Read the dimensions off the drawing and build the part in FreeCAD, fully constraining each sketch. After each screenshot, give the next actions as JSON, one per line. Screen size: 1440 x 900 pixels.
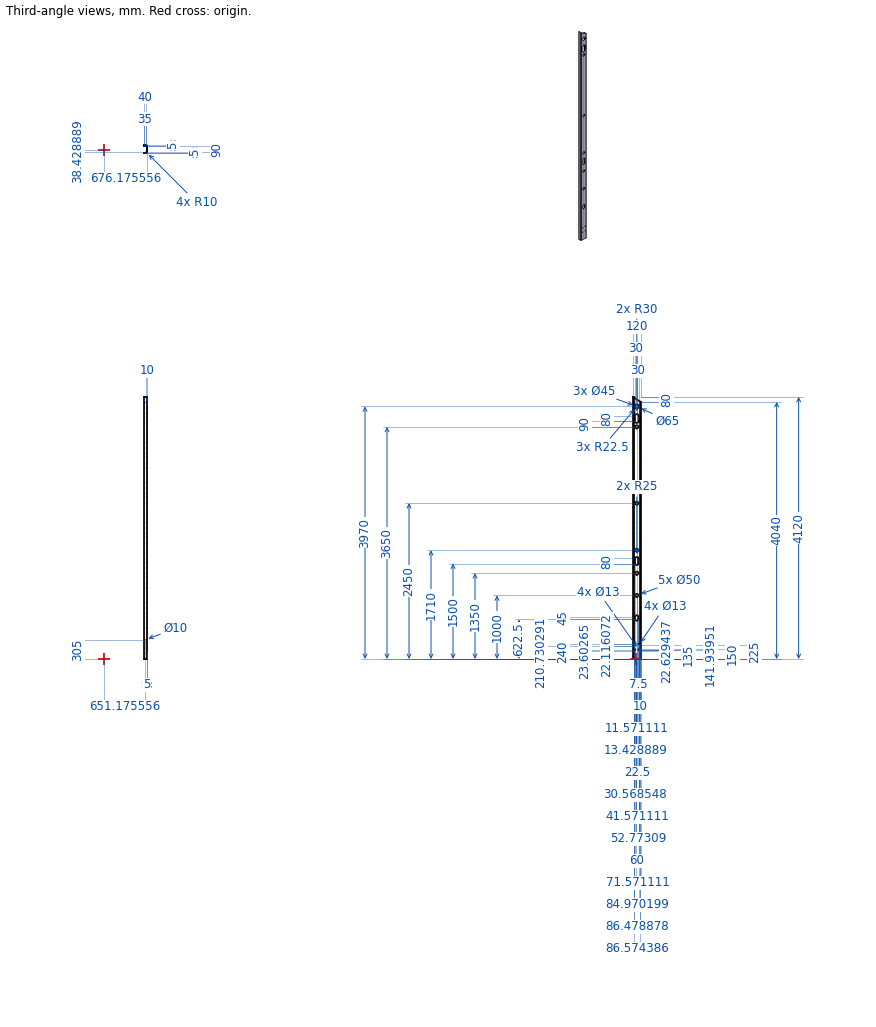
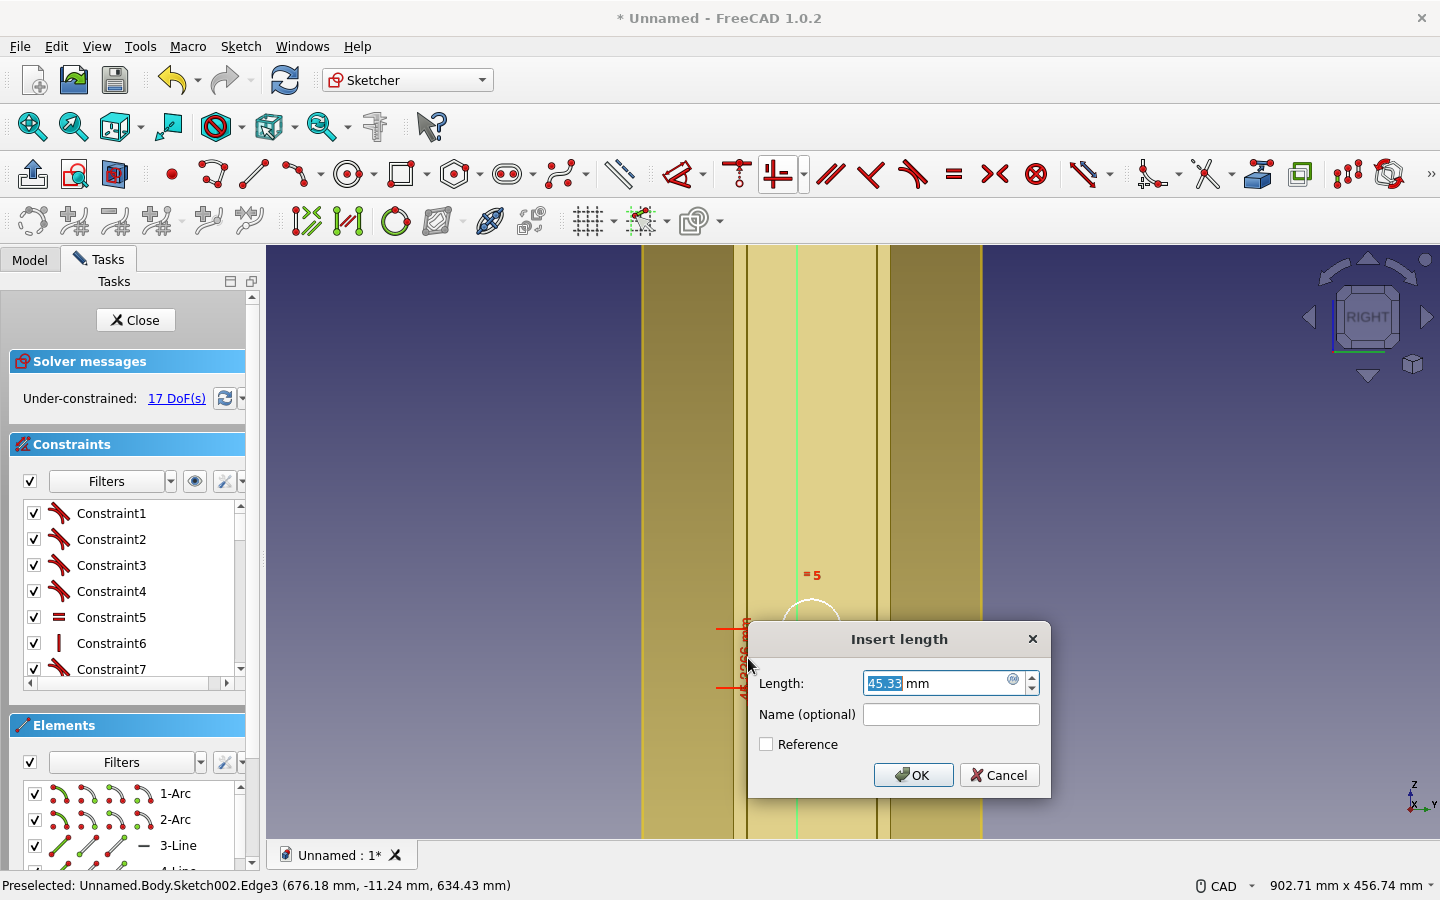
{"action": "type", "text": "45"}
{"action": "key", "text": "Return"}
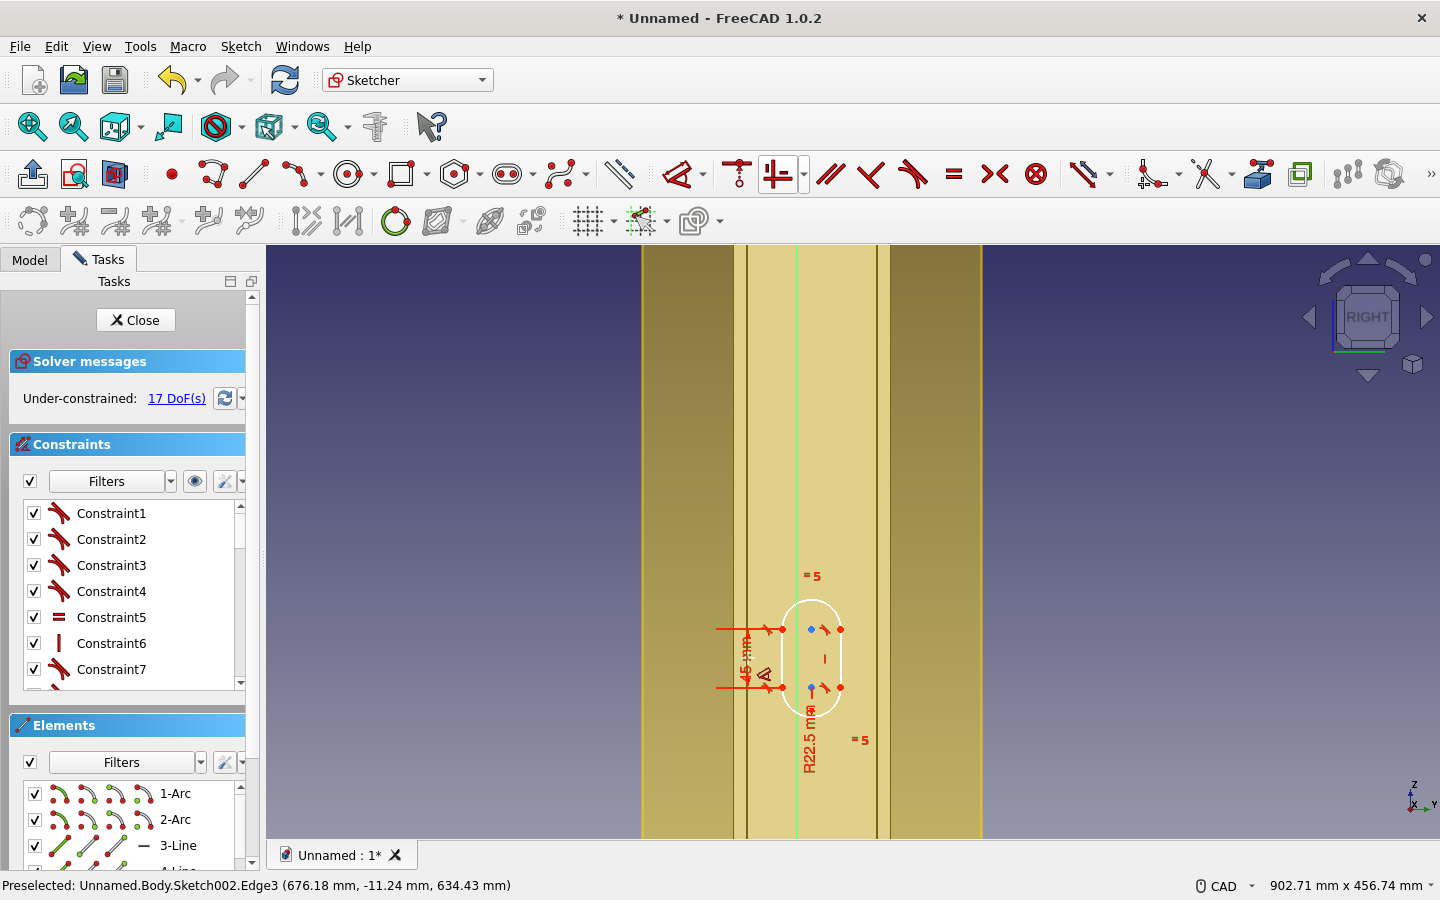
{"action": "scroll", "coordinate": [782, 674], "scroll_direction": "down", "scroll_amount": 13}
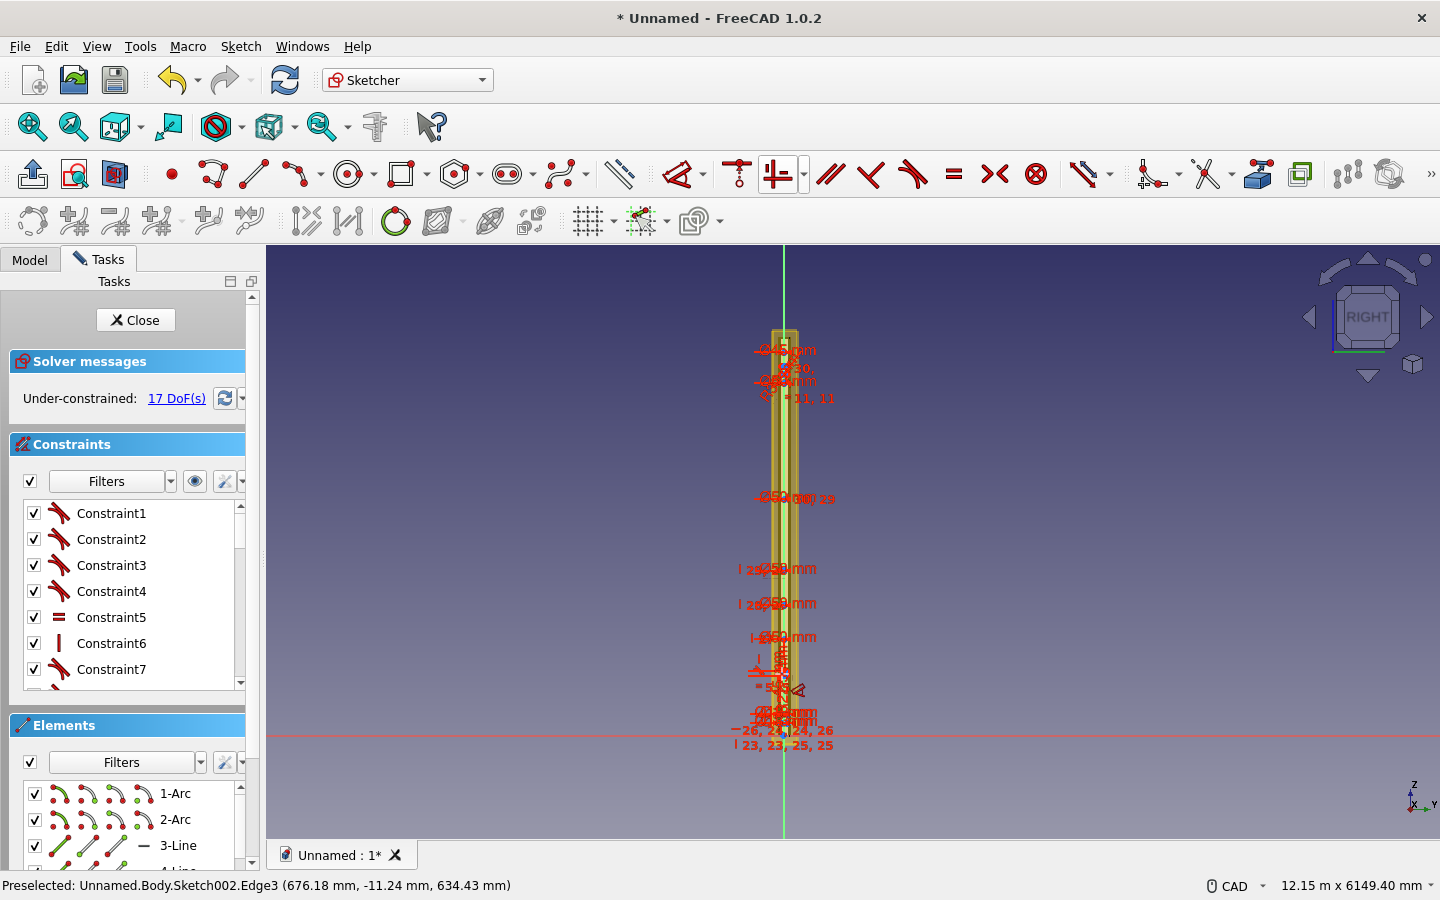
{"action": "scroll", "coordinate": [782, 372], "scroll_direction": "up", "scroll_amount": 11}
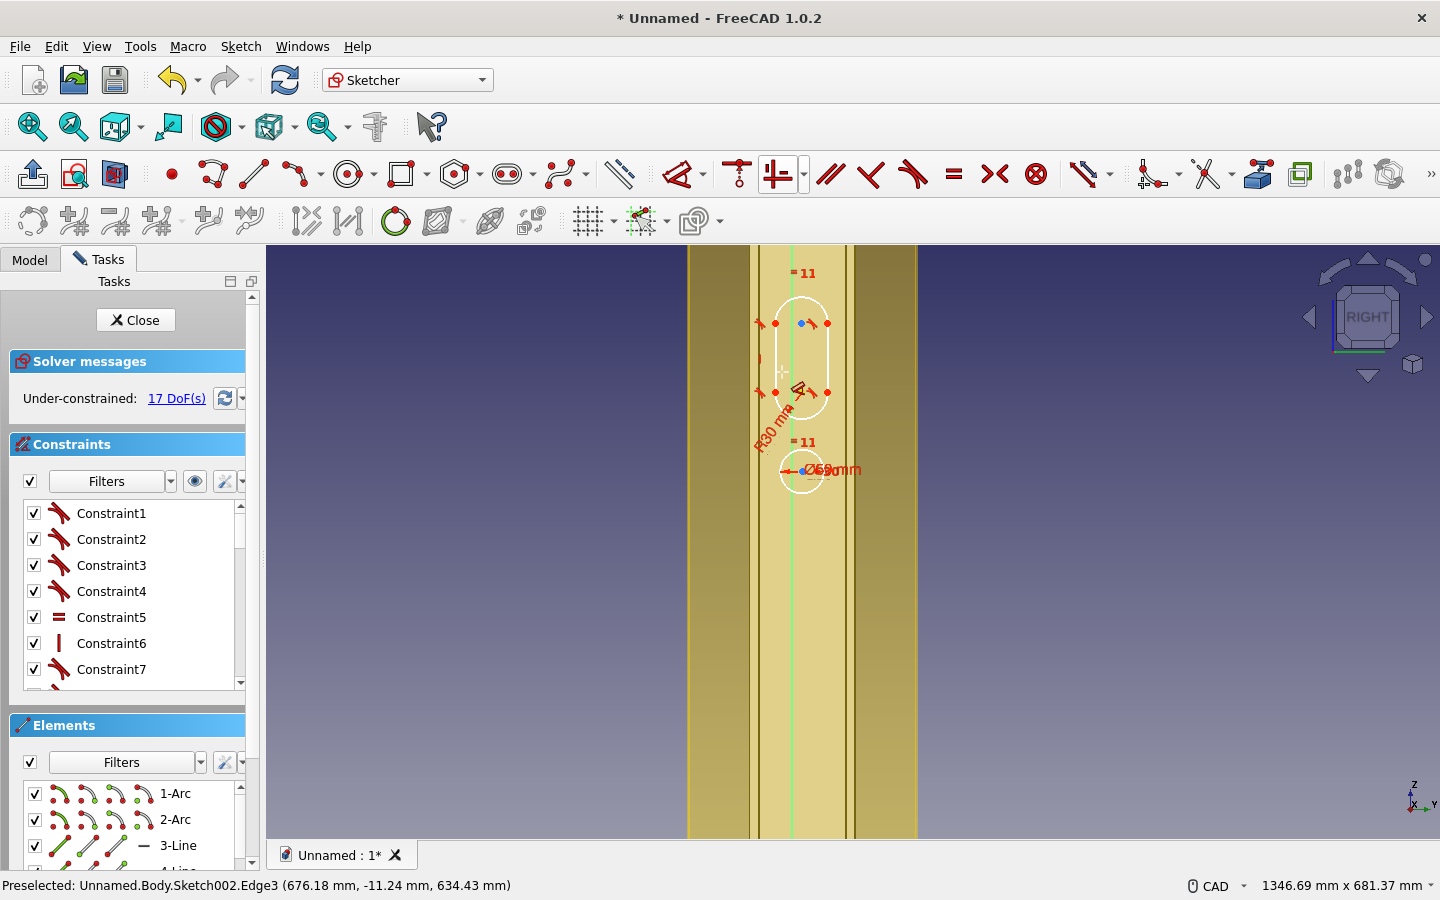
{"action": "left_click", "coordinate": [776, 372]}
{"action": "left_click", "coordinate": [742, 358]}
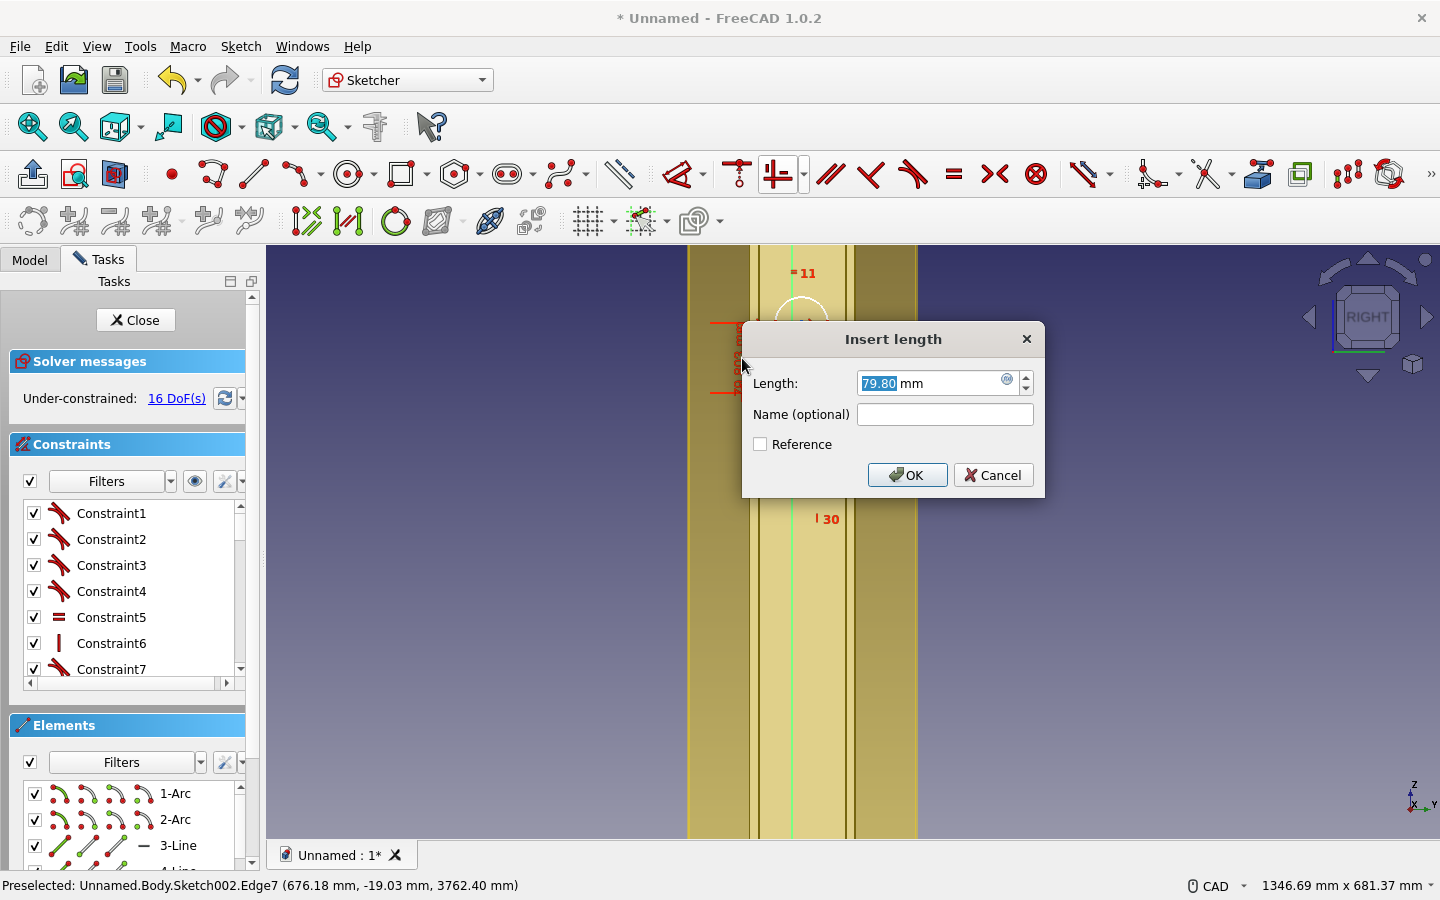
{"action": "type", "text": "80"}
{"action": "key", "text": "Return"}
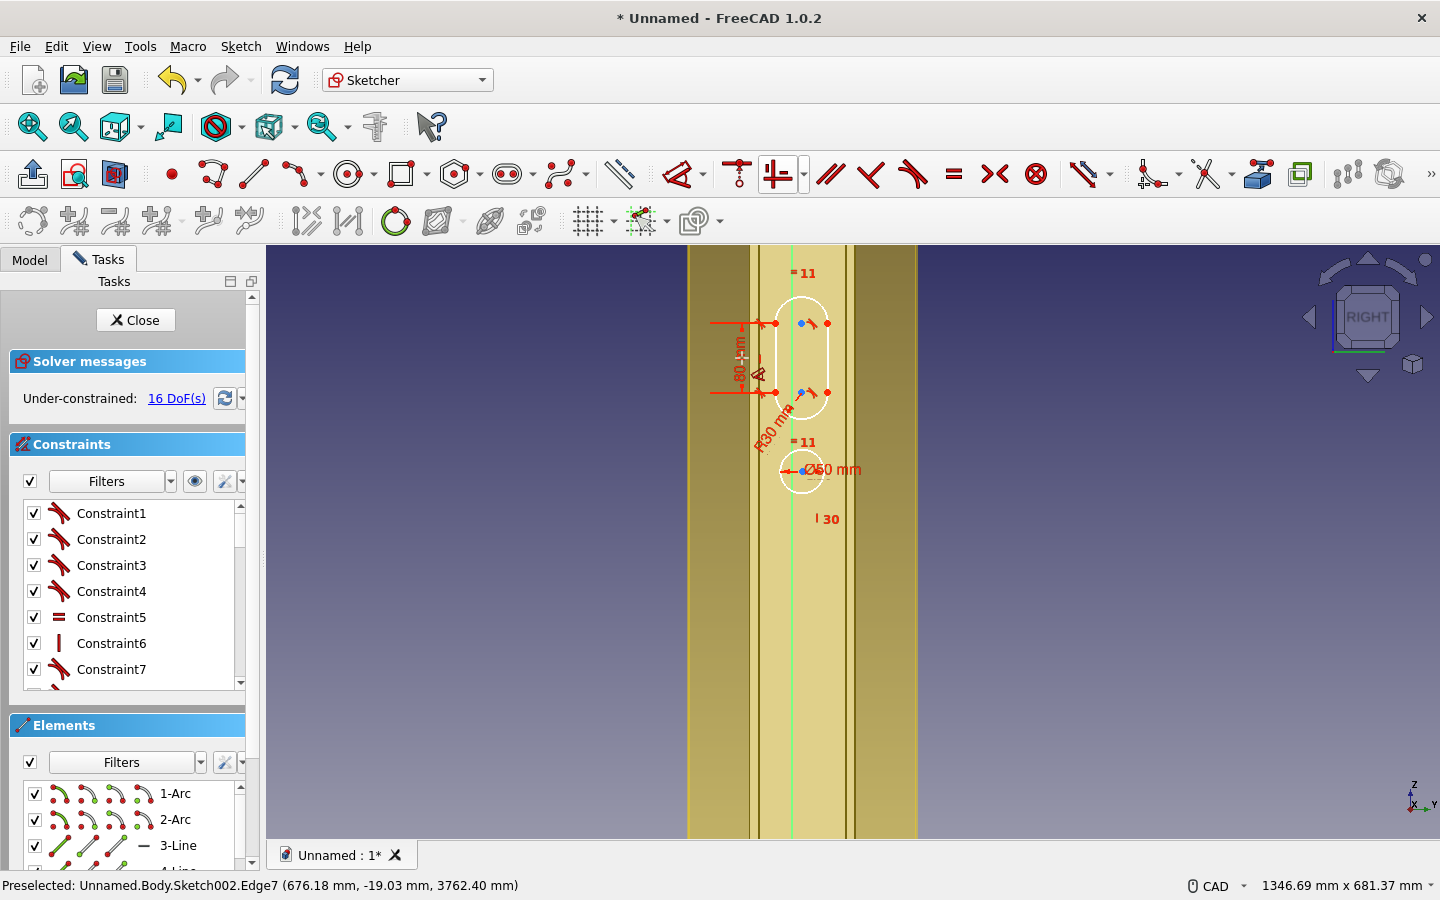
{"action": "scroll", "coordinate": [782, 371], "scroll_direction": "down", "scroll_amount": 11}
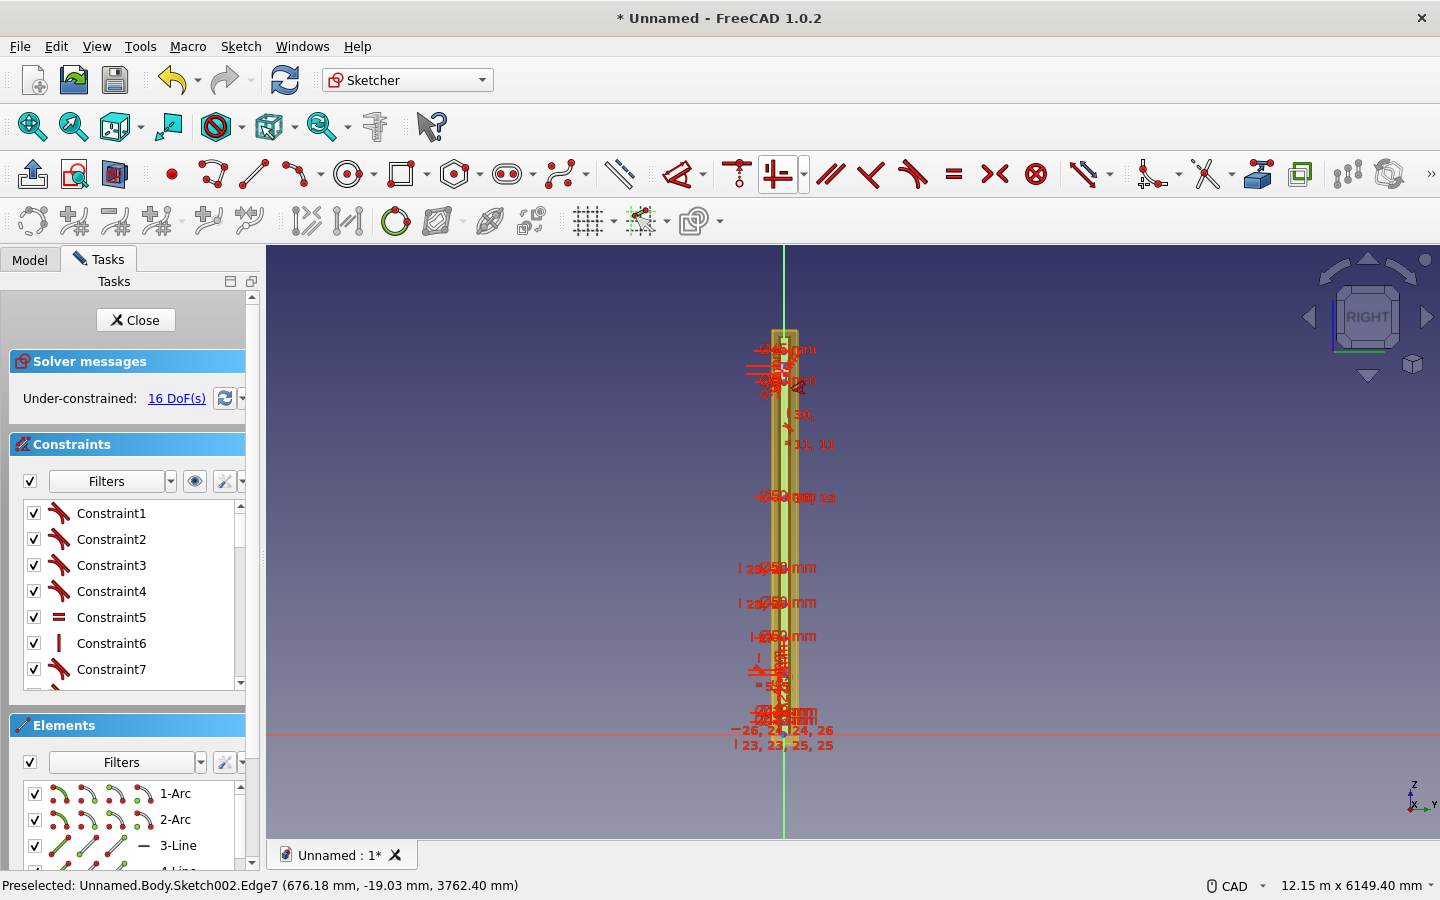
{"action": "scroll", "coordinate": [787, 713], "scroll_direction": "up", "scroll_amount": 4}